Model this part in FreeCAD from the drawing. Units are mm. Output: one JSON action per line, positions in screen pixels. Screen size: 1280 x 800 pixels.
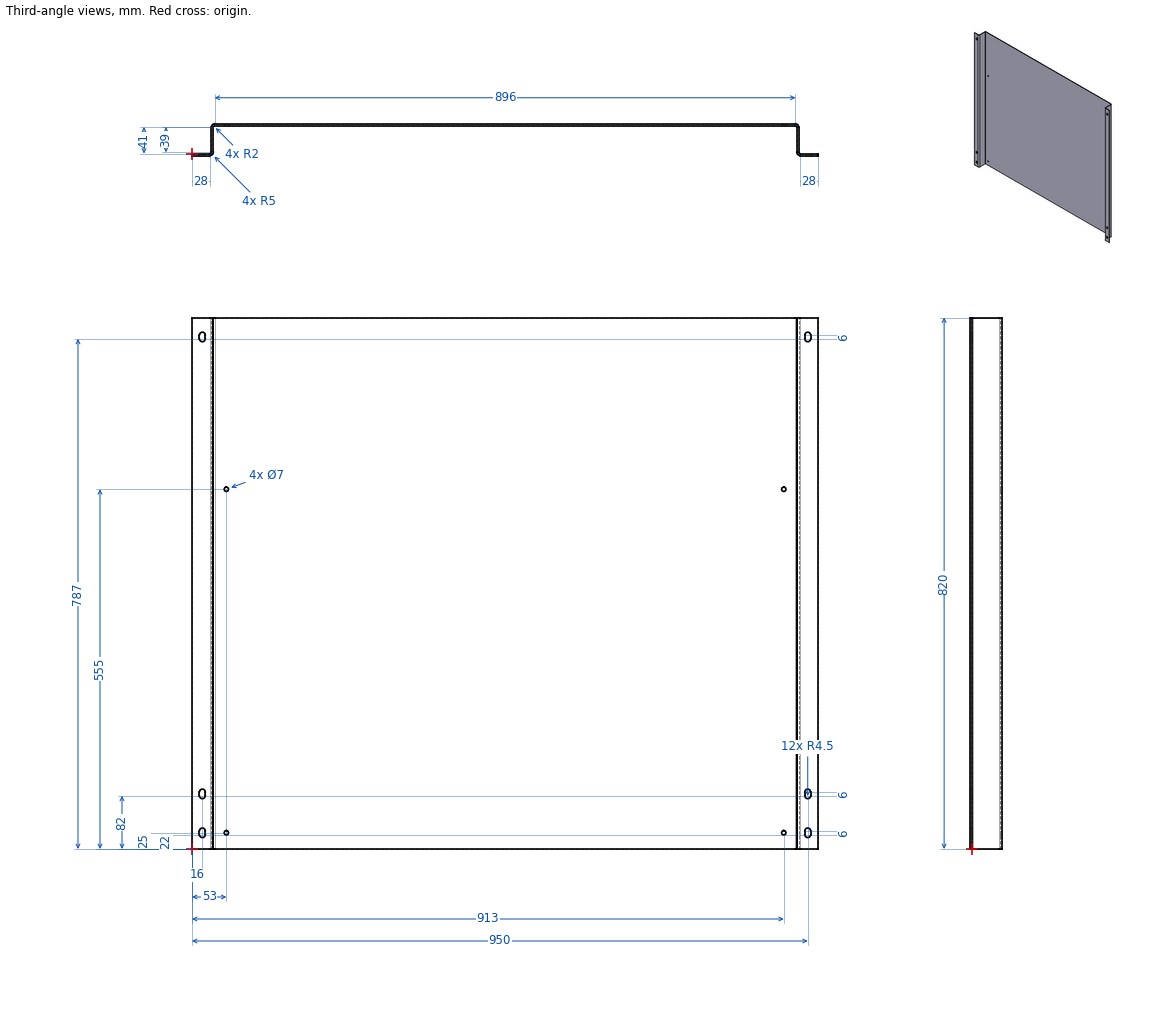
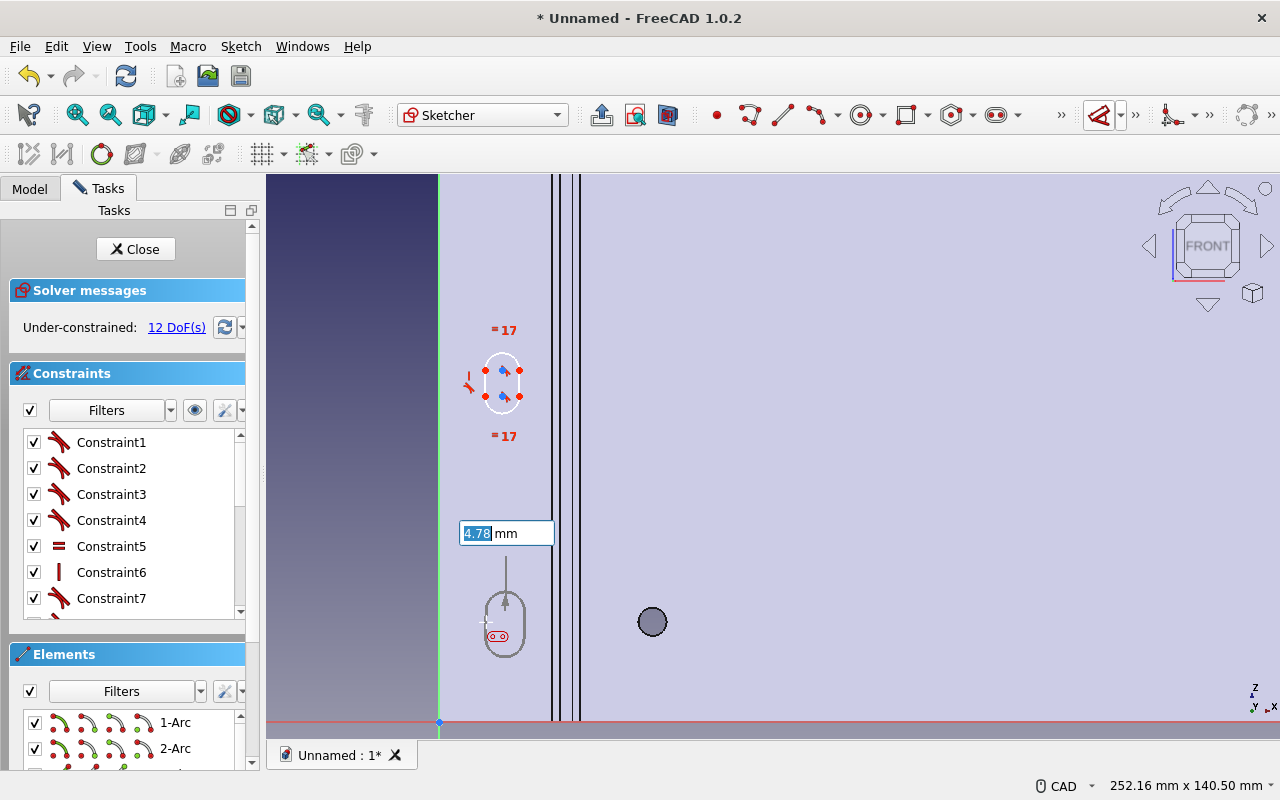
{"action": "left_click", "coordinate": [486, 622]}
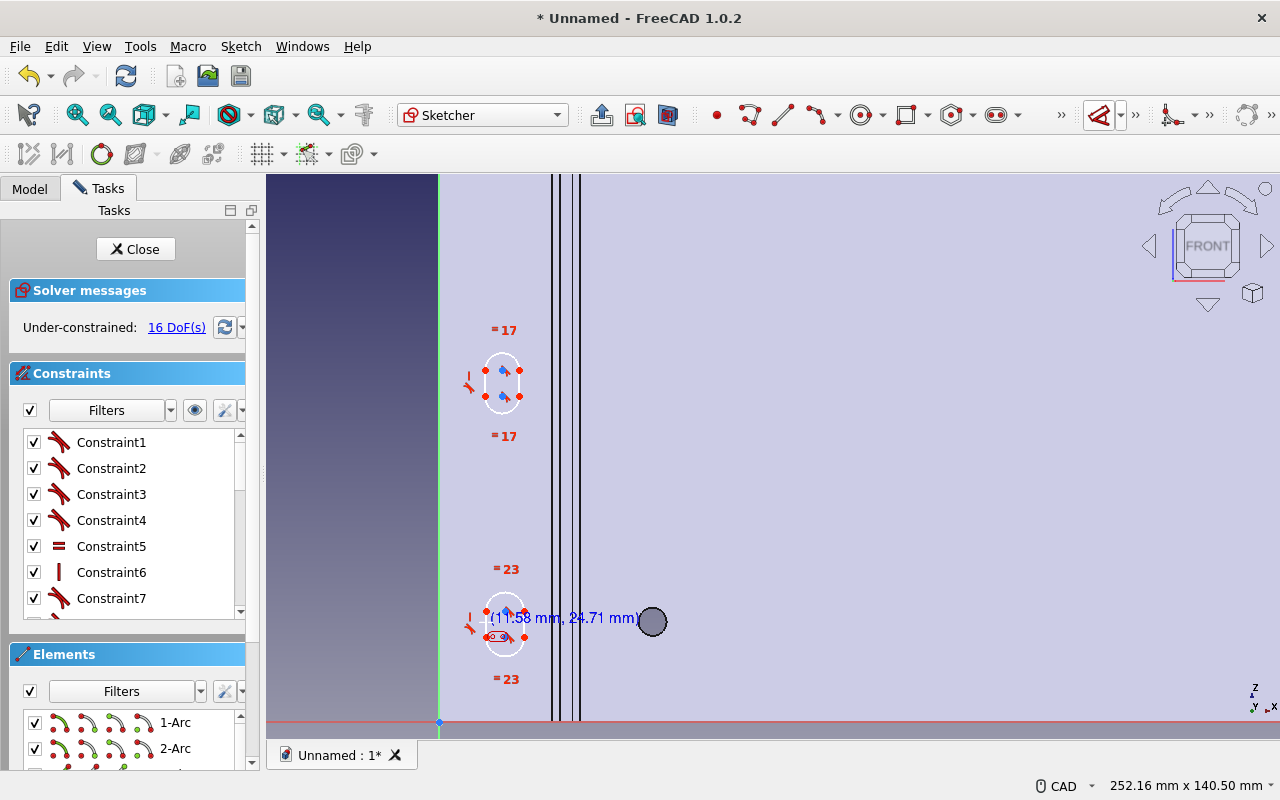
{"action": "scroll", "coordinate": [498, 623], "scroll_direction": "down", "scroll_amount": 11}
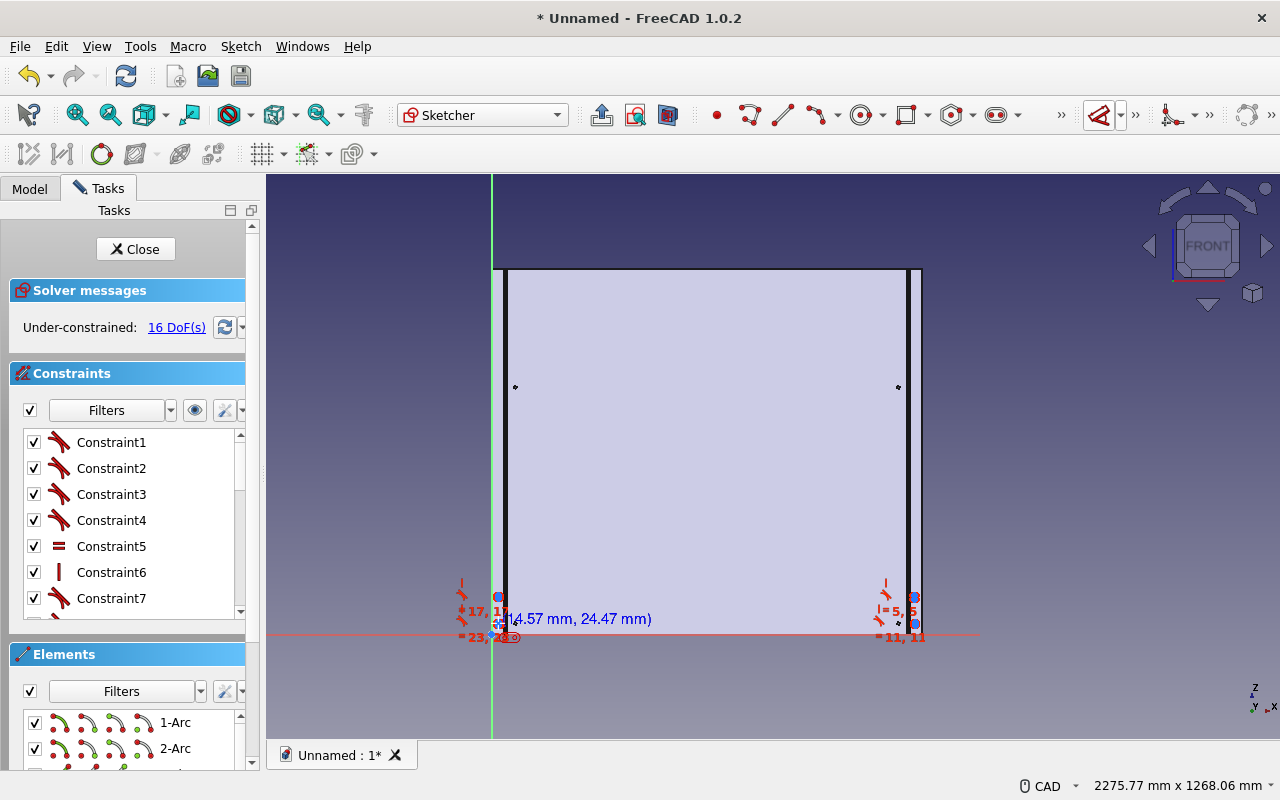
{"action": "scroll", "coordinate": [915, 284], "scroll_direction": "up", "scroll_amount": 13}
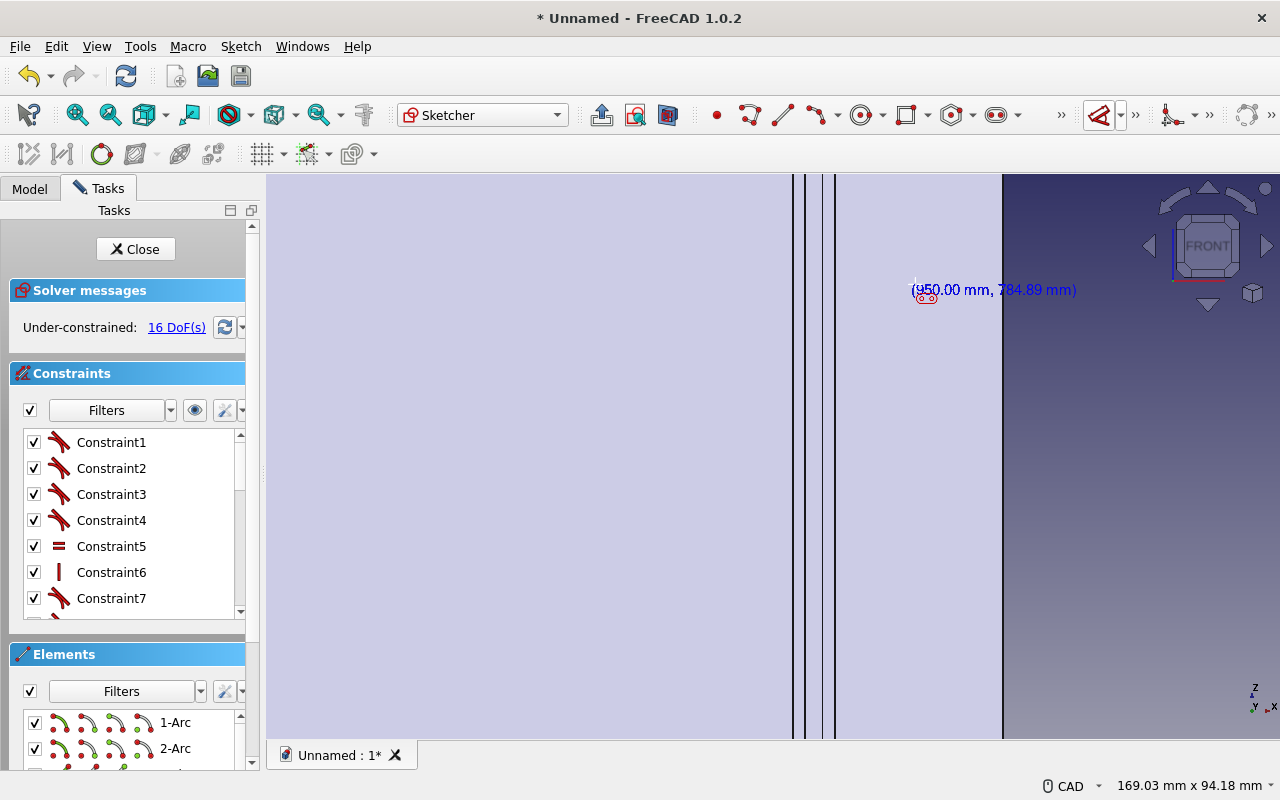
{"action": "scroll", "coordinate": [916, 284], "scroll_direction": "down", "scroll_amount": 13}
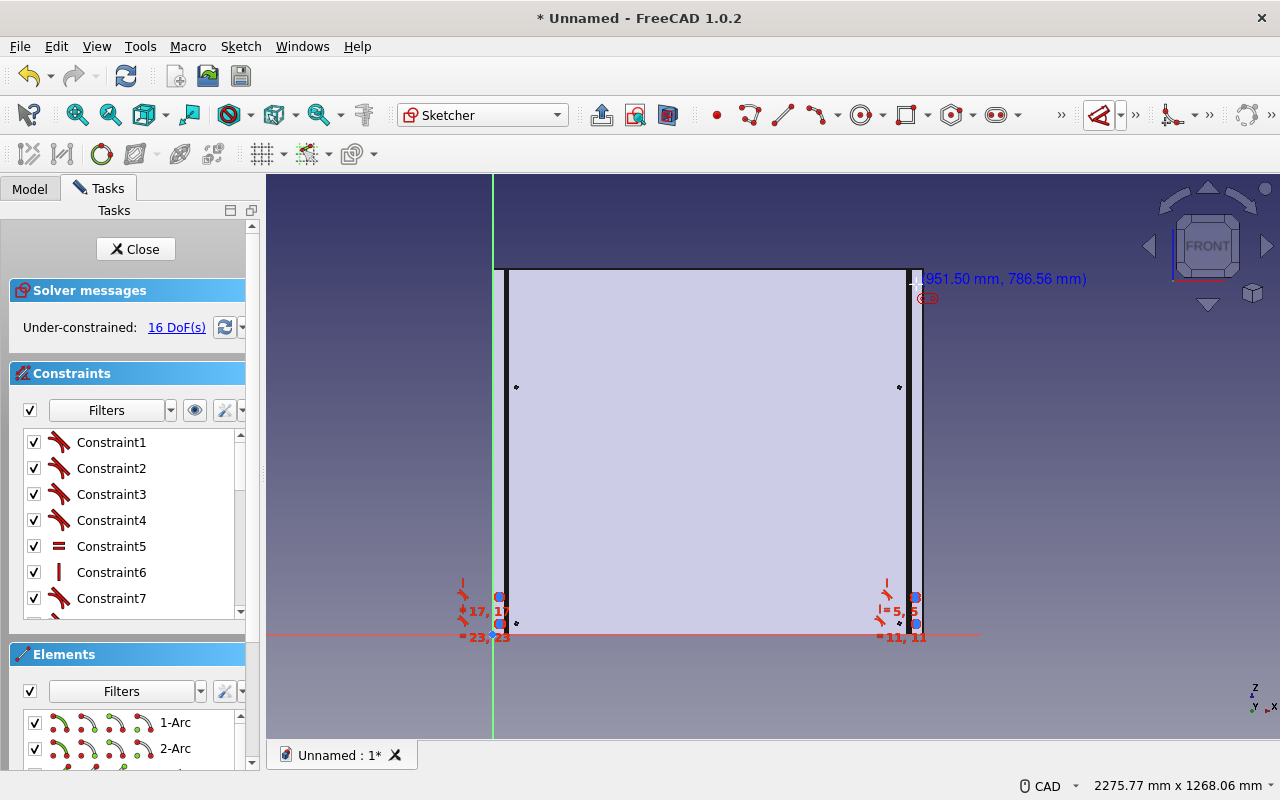
{"action": "left_click", "coordinate": [916, 284]}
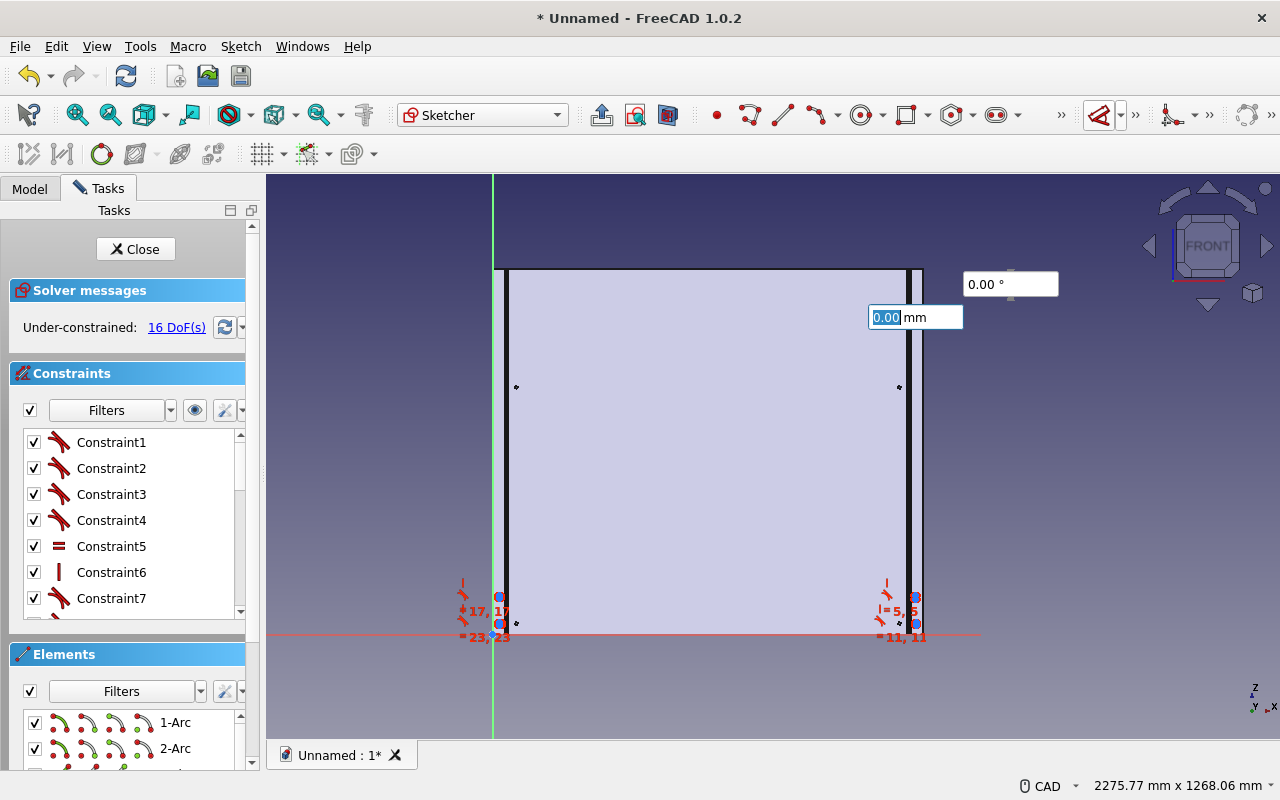
{"action": "scroll", "coordinate": [916, 281], "scroll_direction": "up", "scroll_amount": 9}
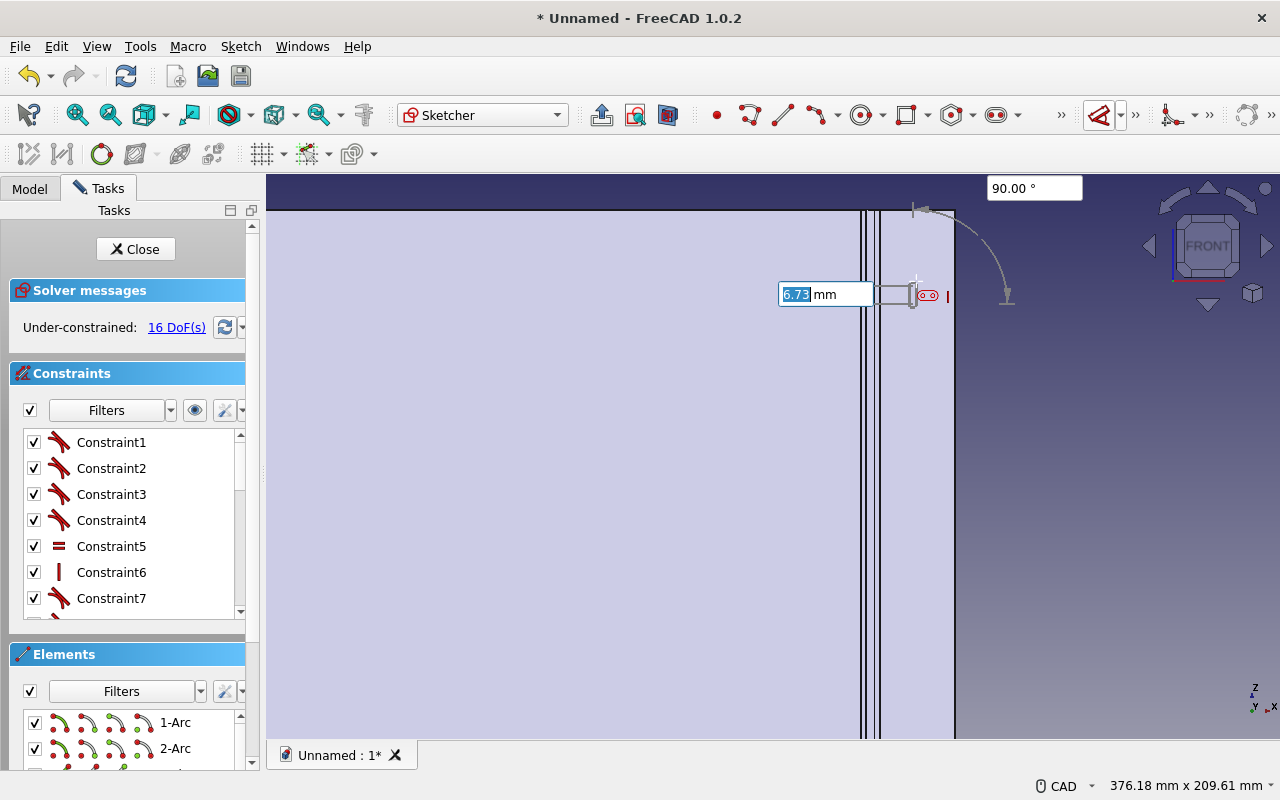
{"action": "left_click", "coordinate": [913, 282]}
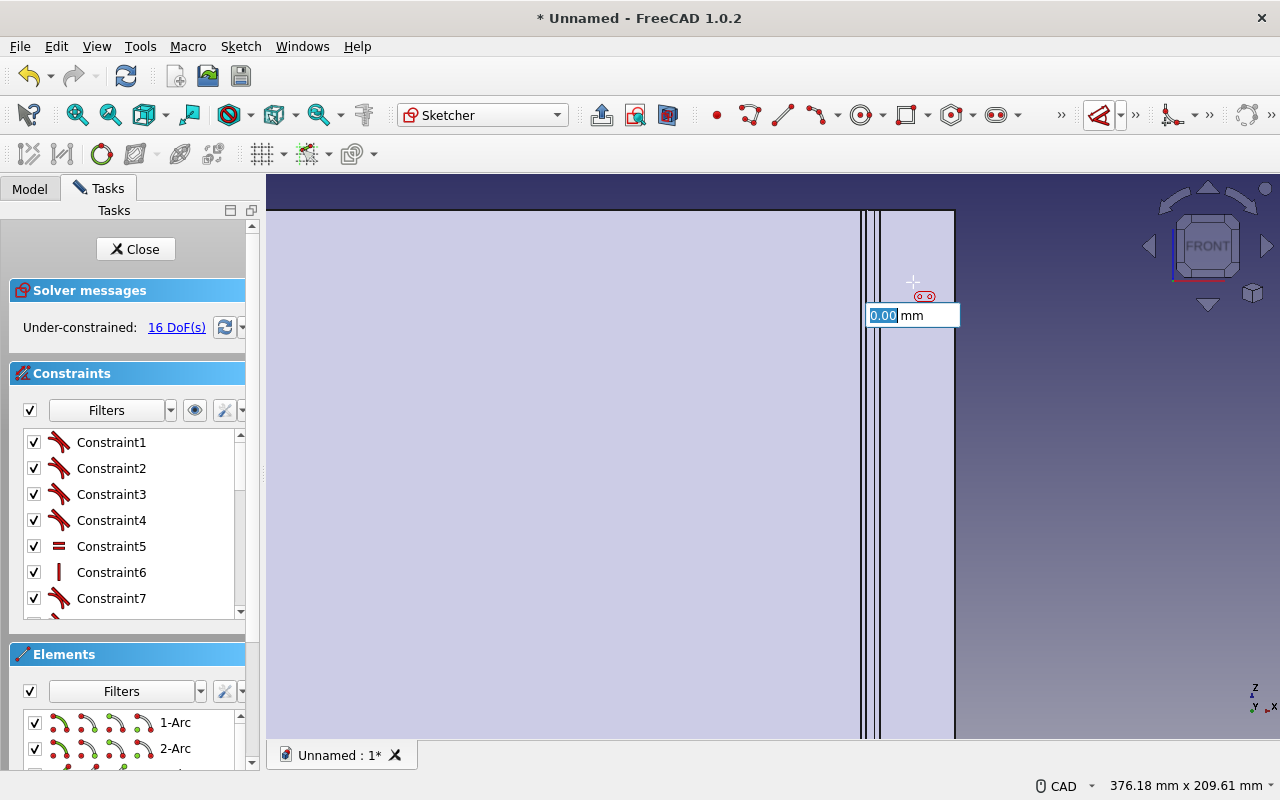
{"action": "scroll", "coordinate": [924, 290], "scroll_direction": "up", "scroll_amount": 2}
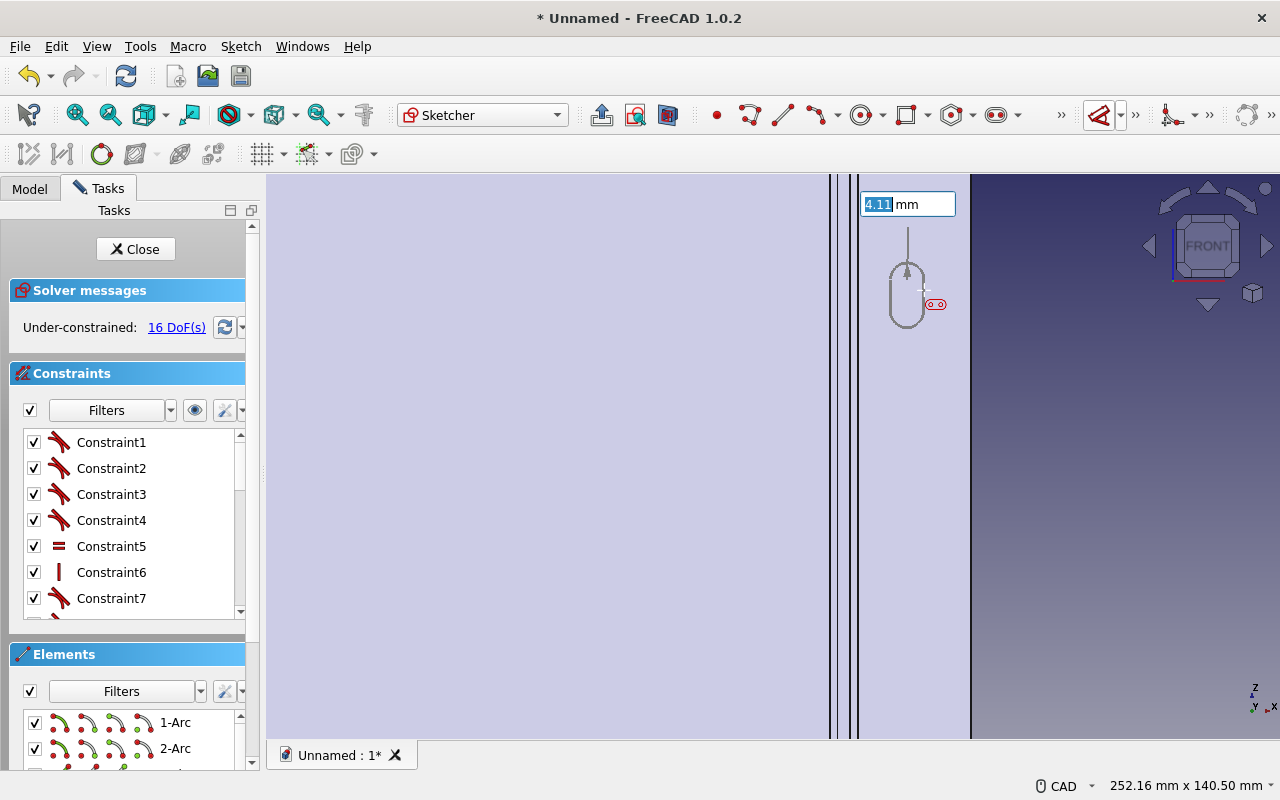
{"action": "left_click", "coordinate": [924, 291]}